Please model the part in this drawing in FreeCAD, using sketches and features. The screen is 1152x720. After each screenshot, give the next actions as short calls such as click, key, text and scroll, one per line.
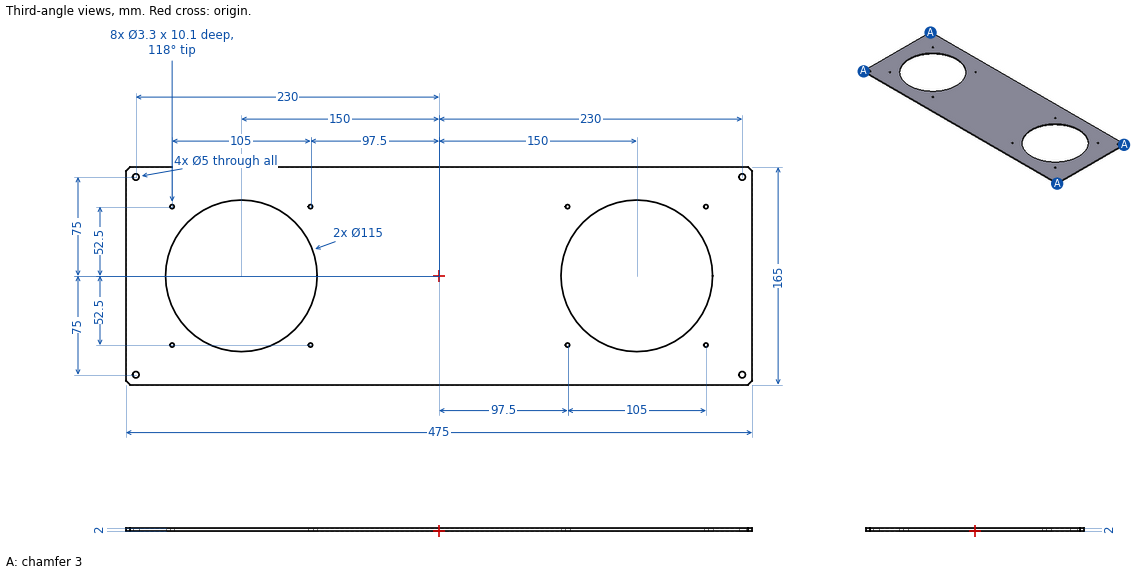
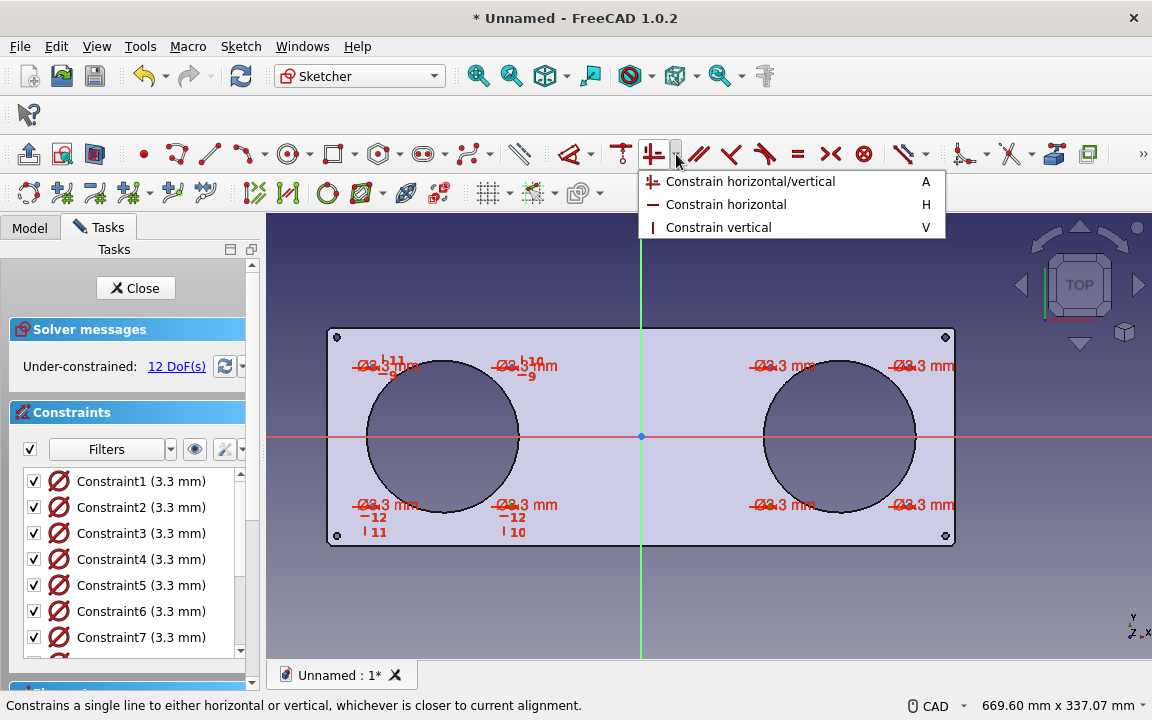
click(792, 204)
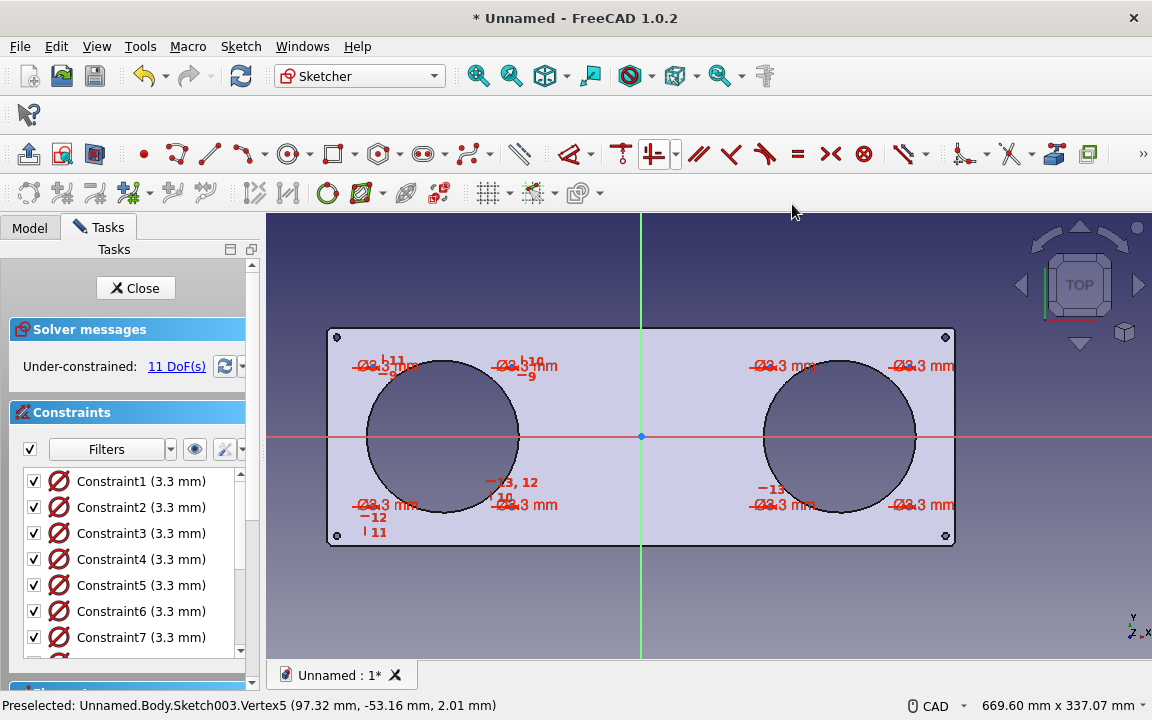
click(770, 507)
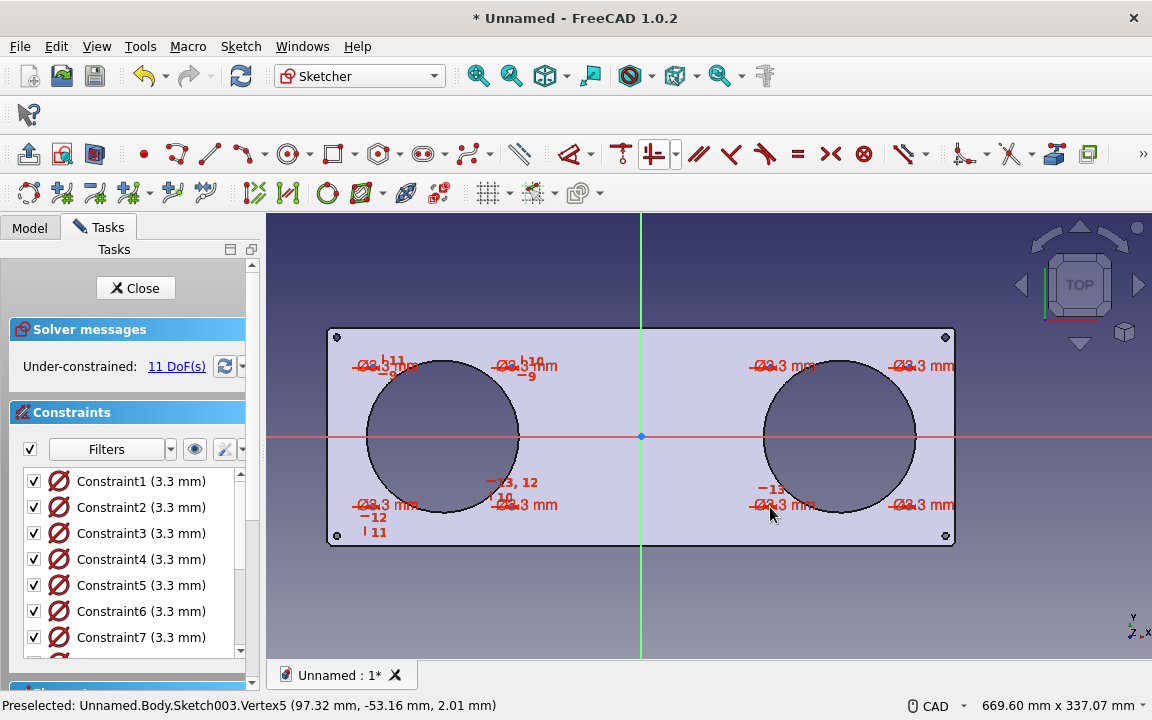
click(909, 507)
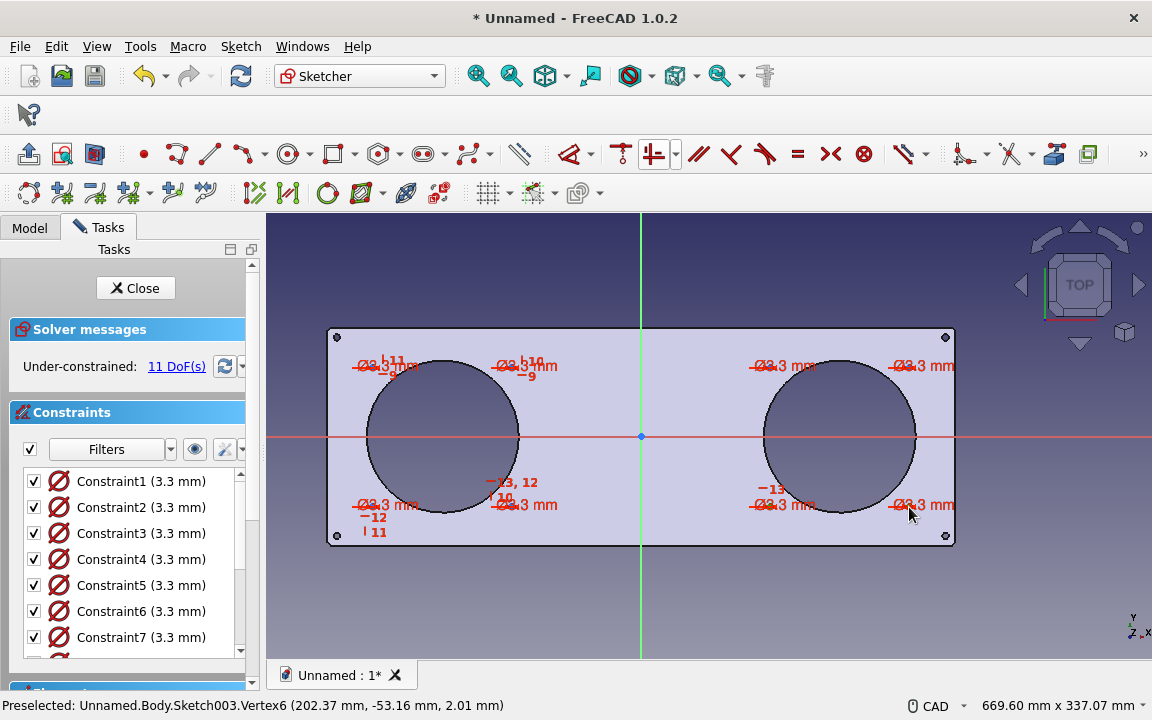
key(h)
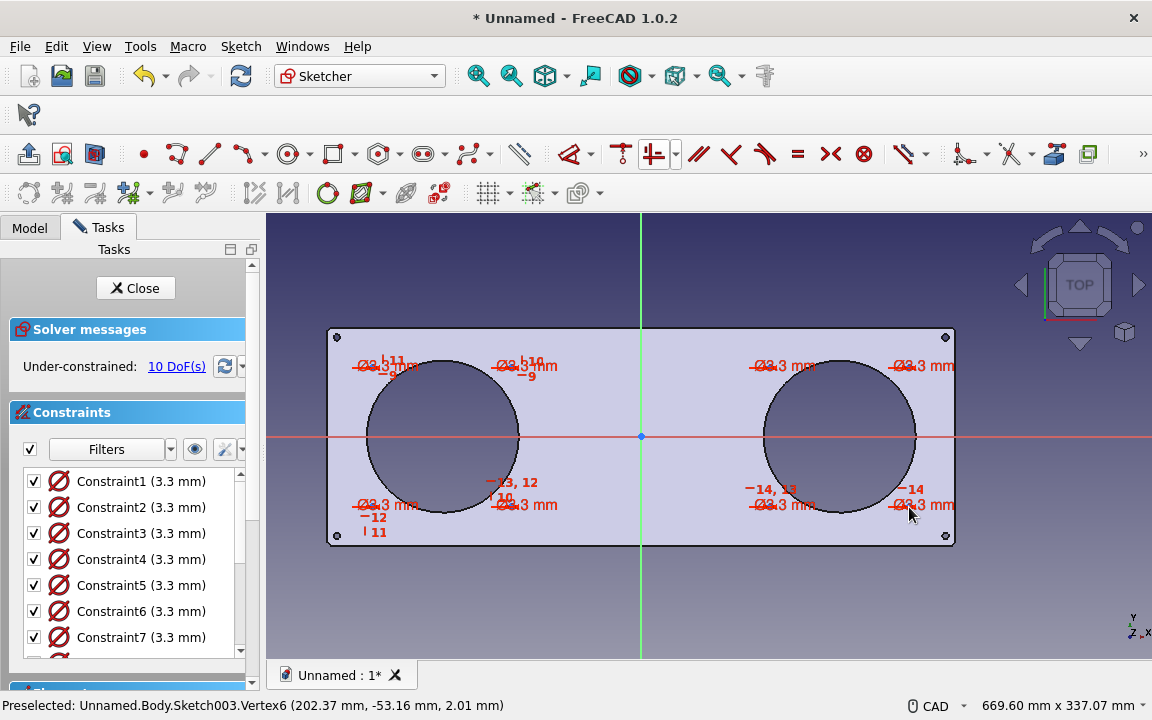
click(909, 507)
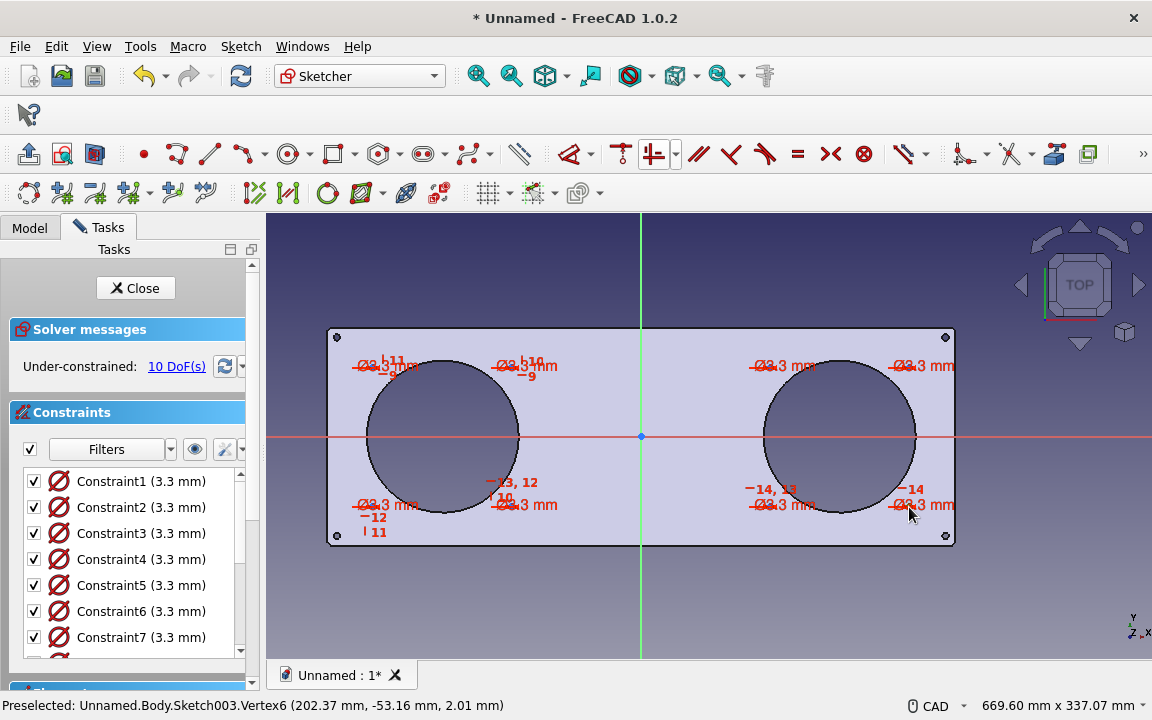
click(909, 368)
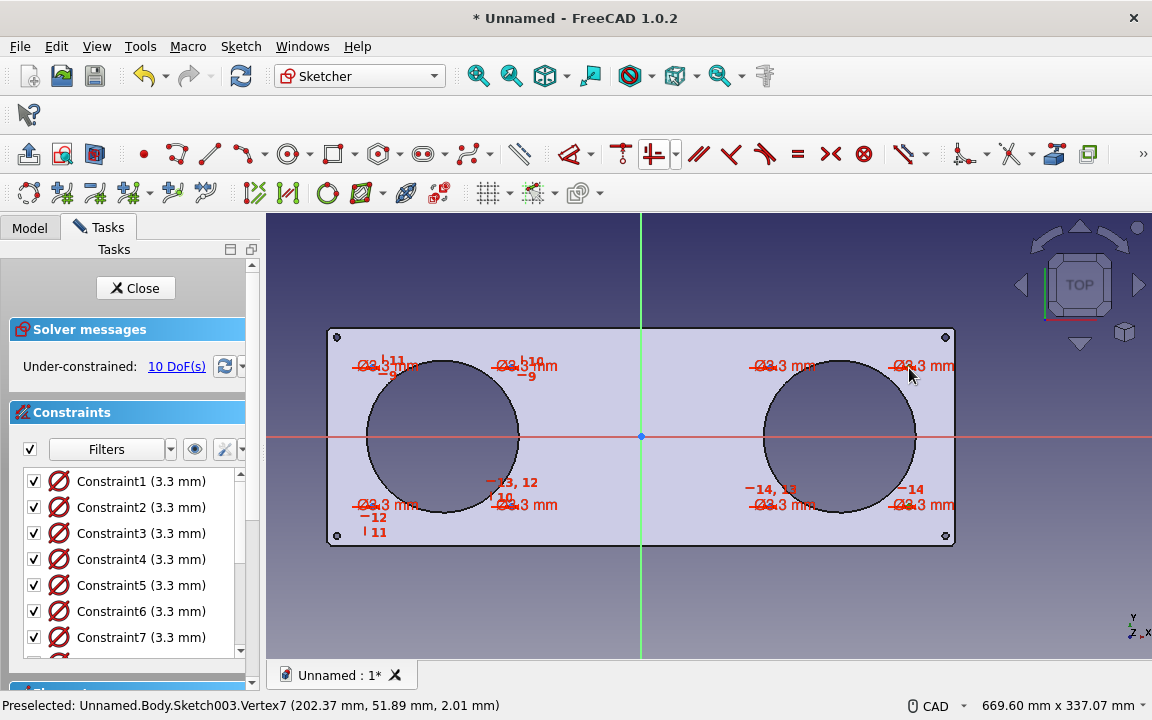
key(v)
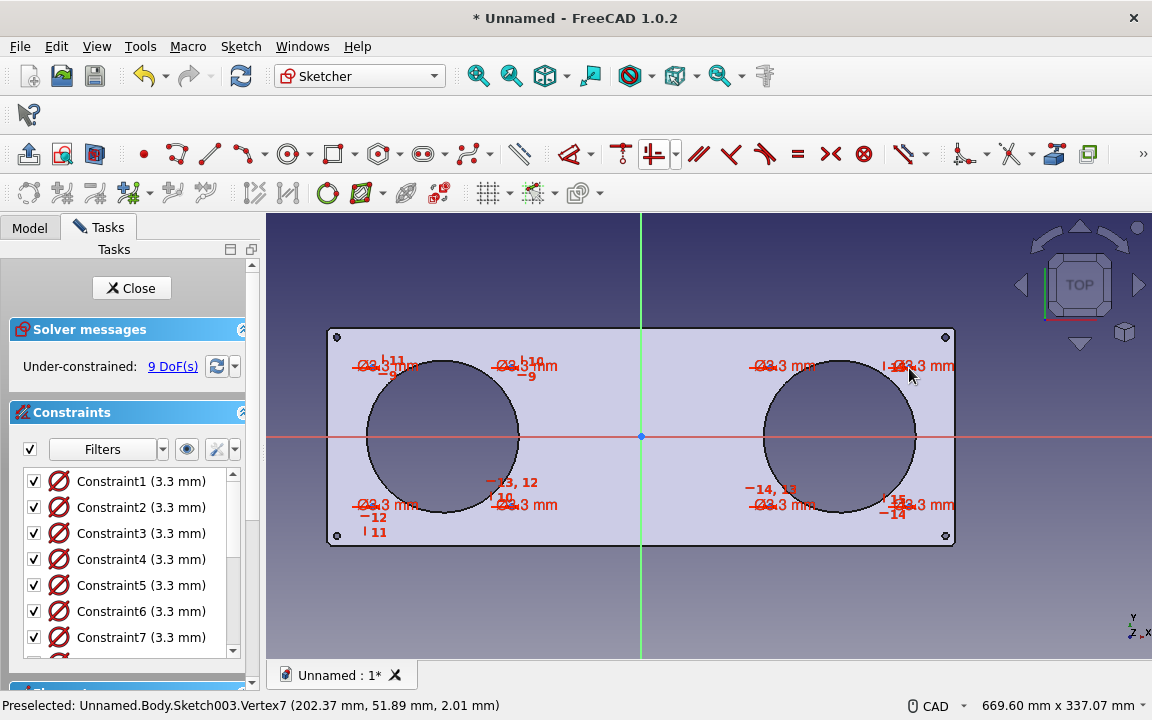
click(512, 368)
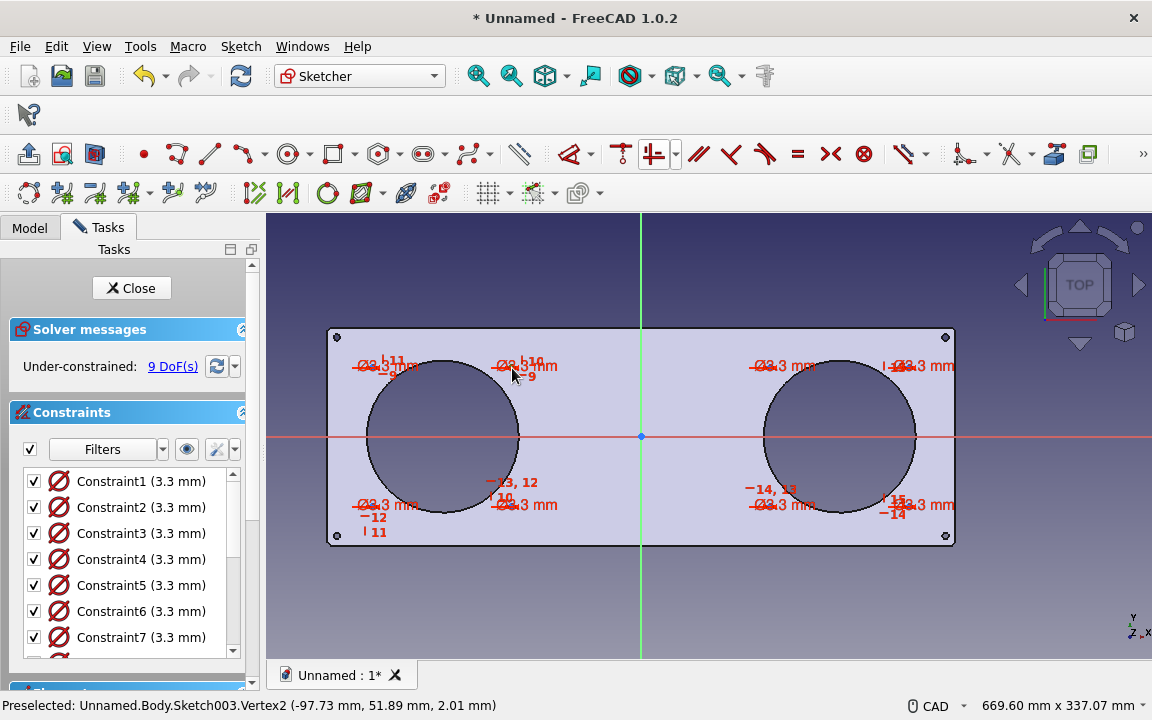
click(909, 368)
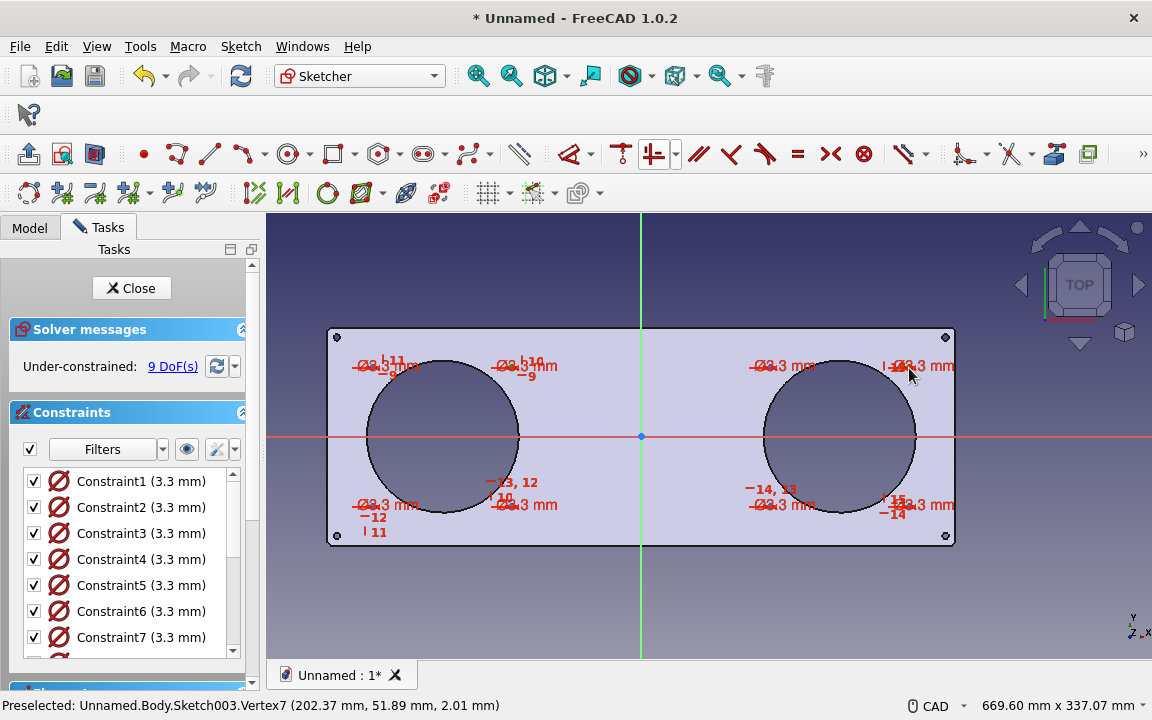
key(h)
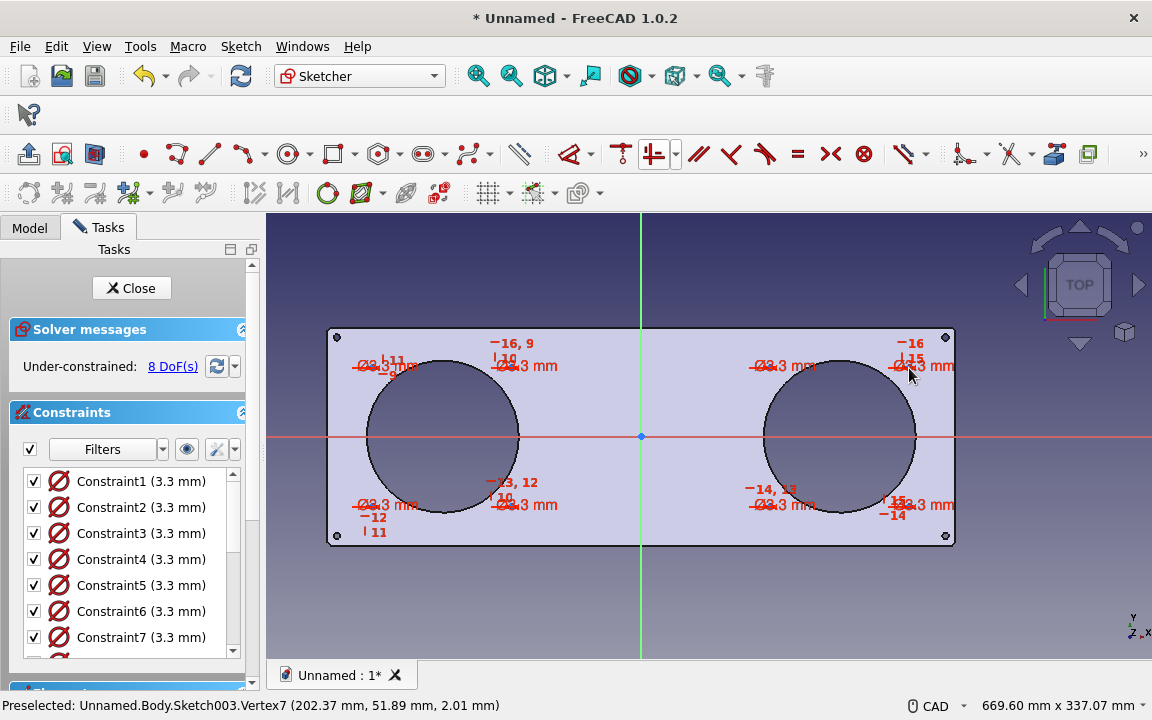
click(770, 507)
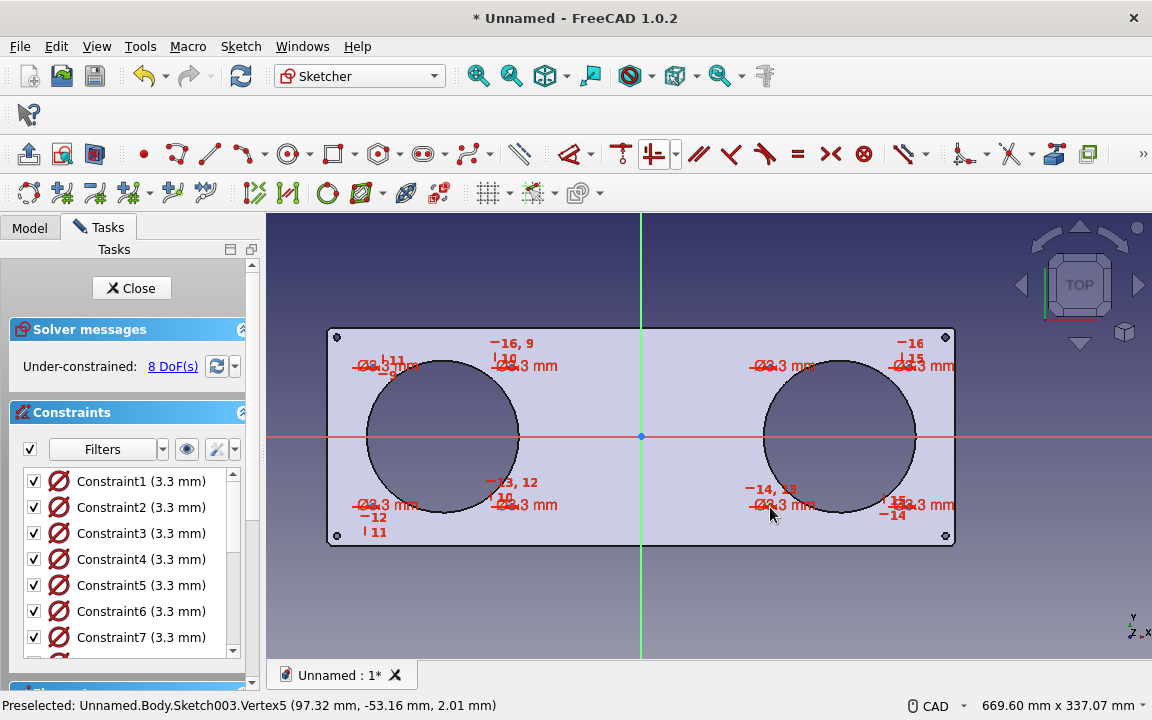
click(770, 368)